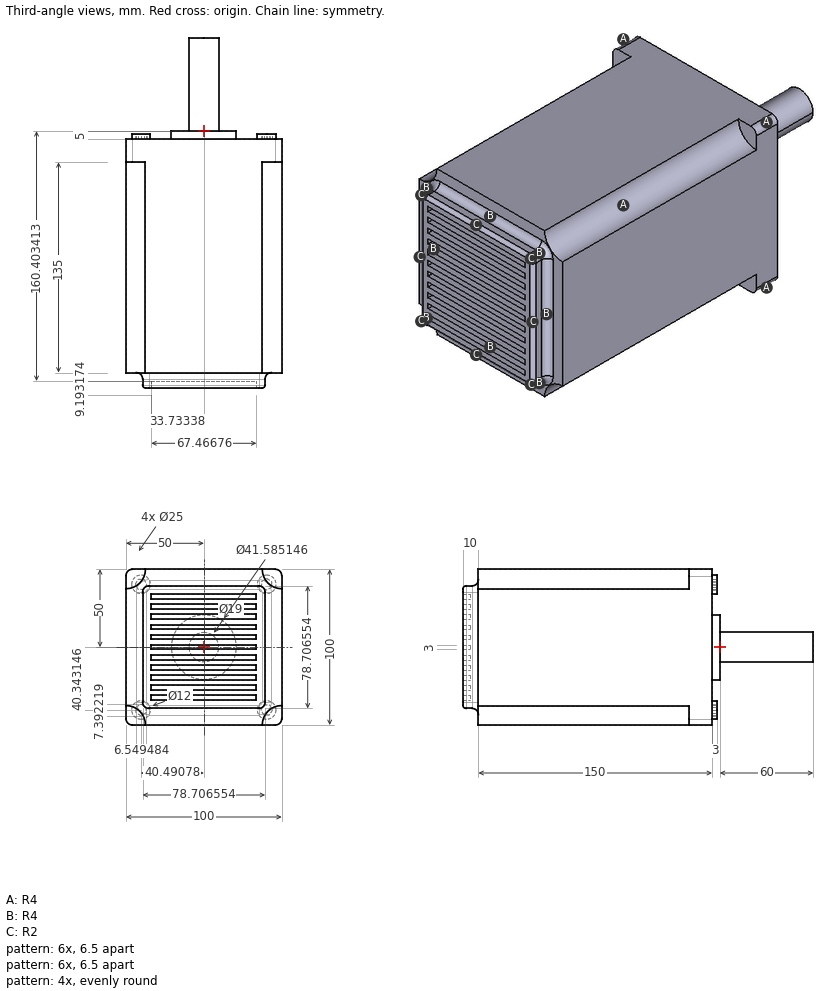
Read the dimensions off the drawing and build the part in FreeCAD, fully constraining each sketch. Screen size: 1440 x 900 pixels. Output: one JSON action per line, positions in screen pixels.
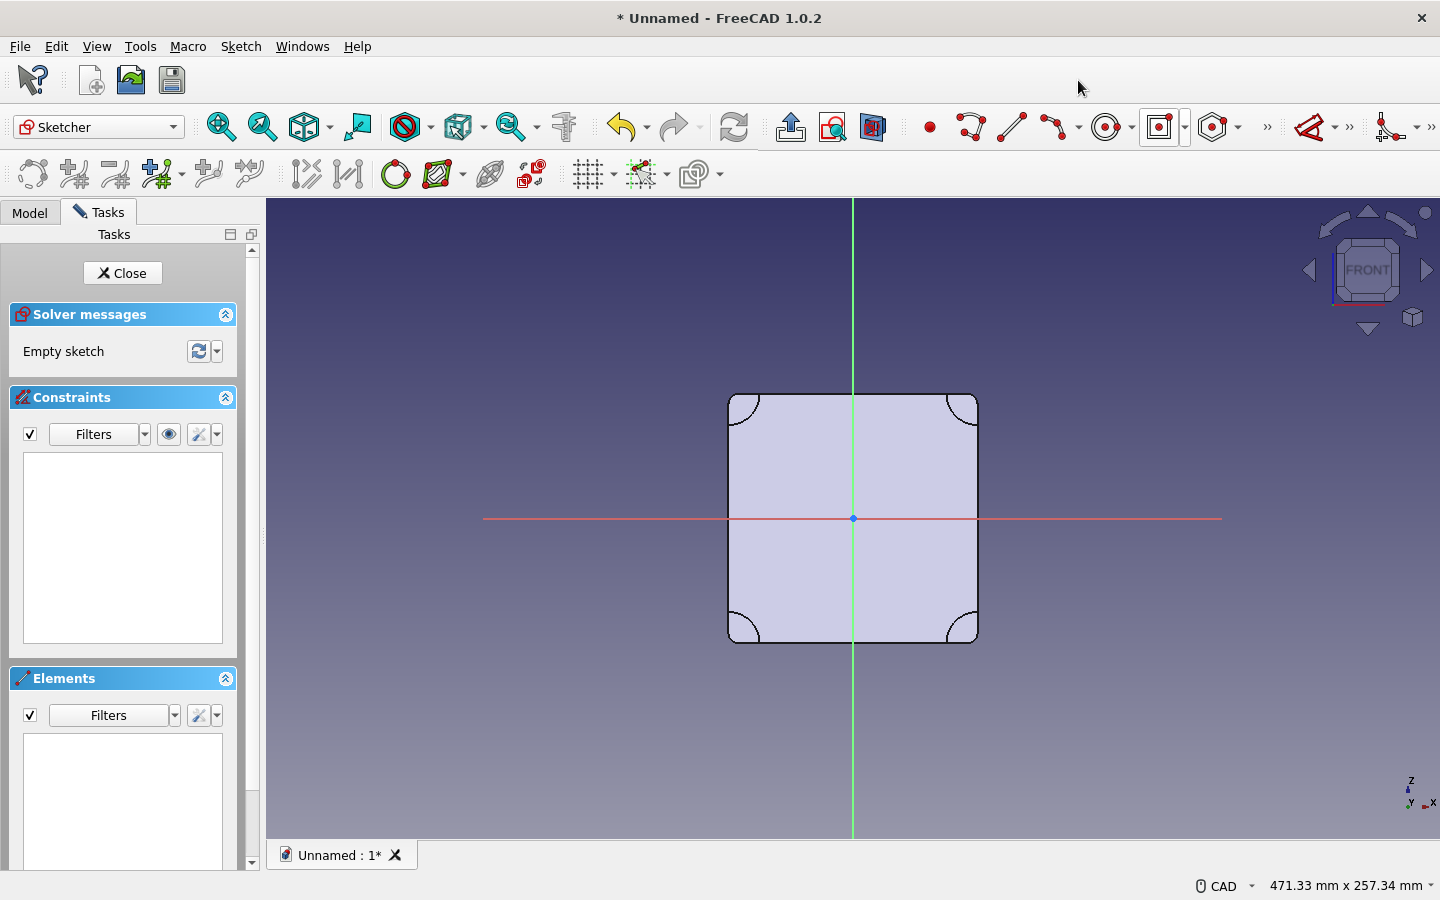
{"action": "scroll", "coordinate": [909, 518], "scroll_direction": "up", "scroll_amount": 4}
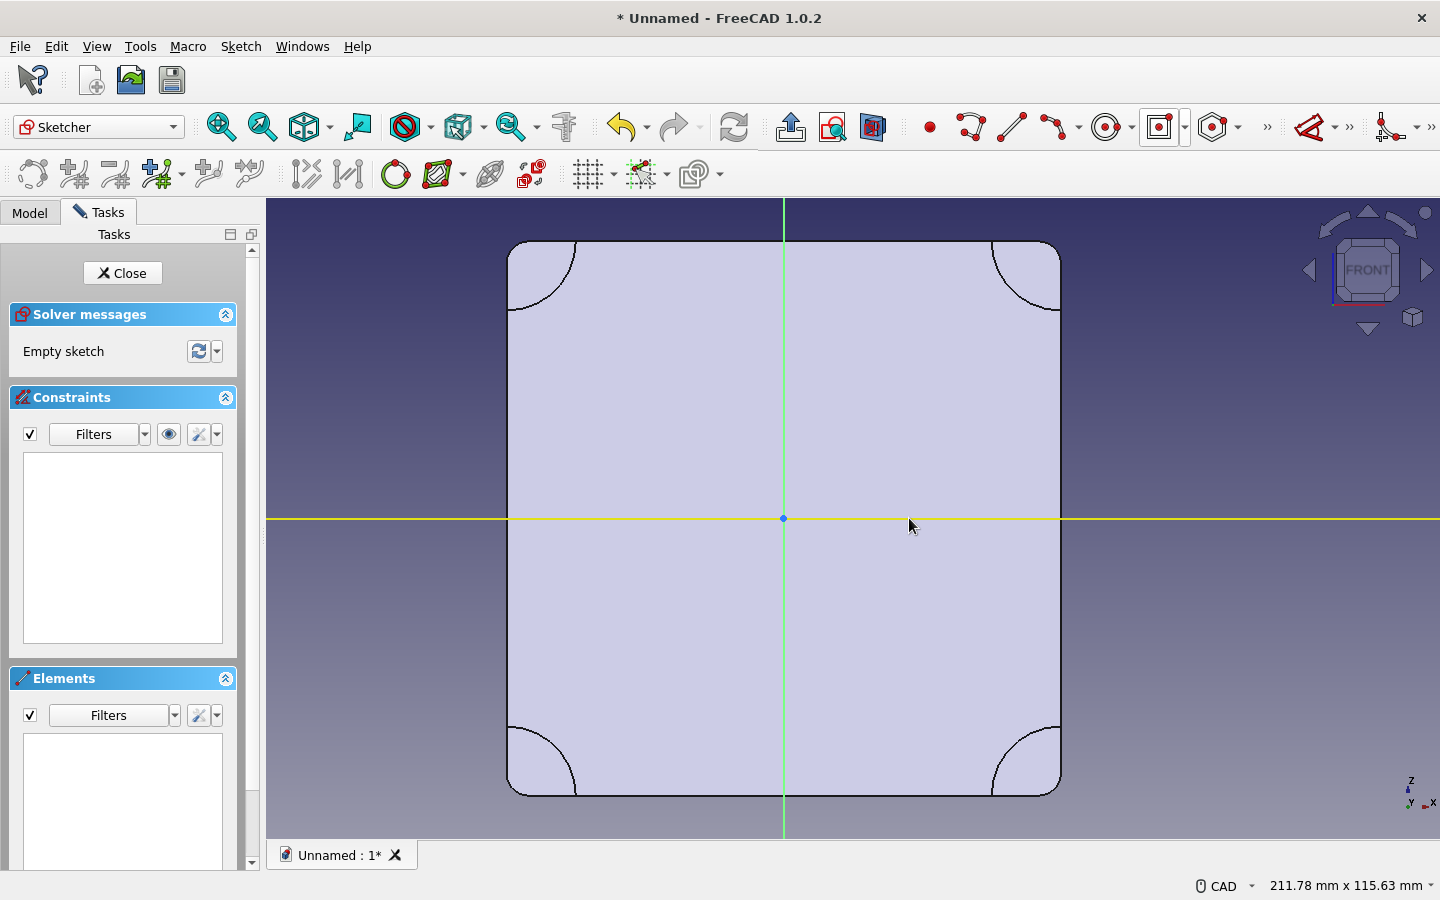
{"action": "left_click", "coordinate": [1158, 128]}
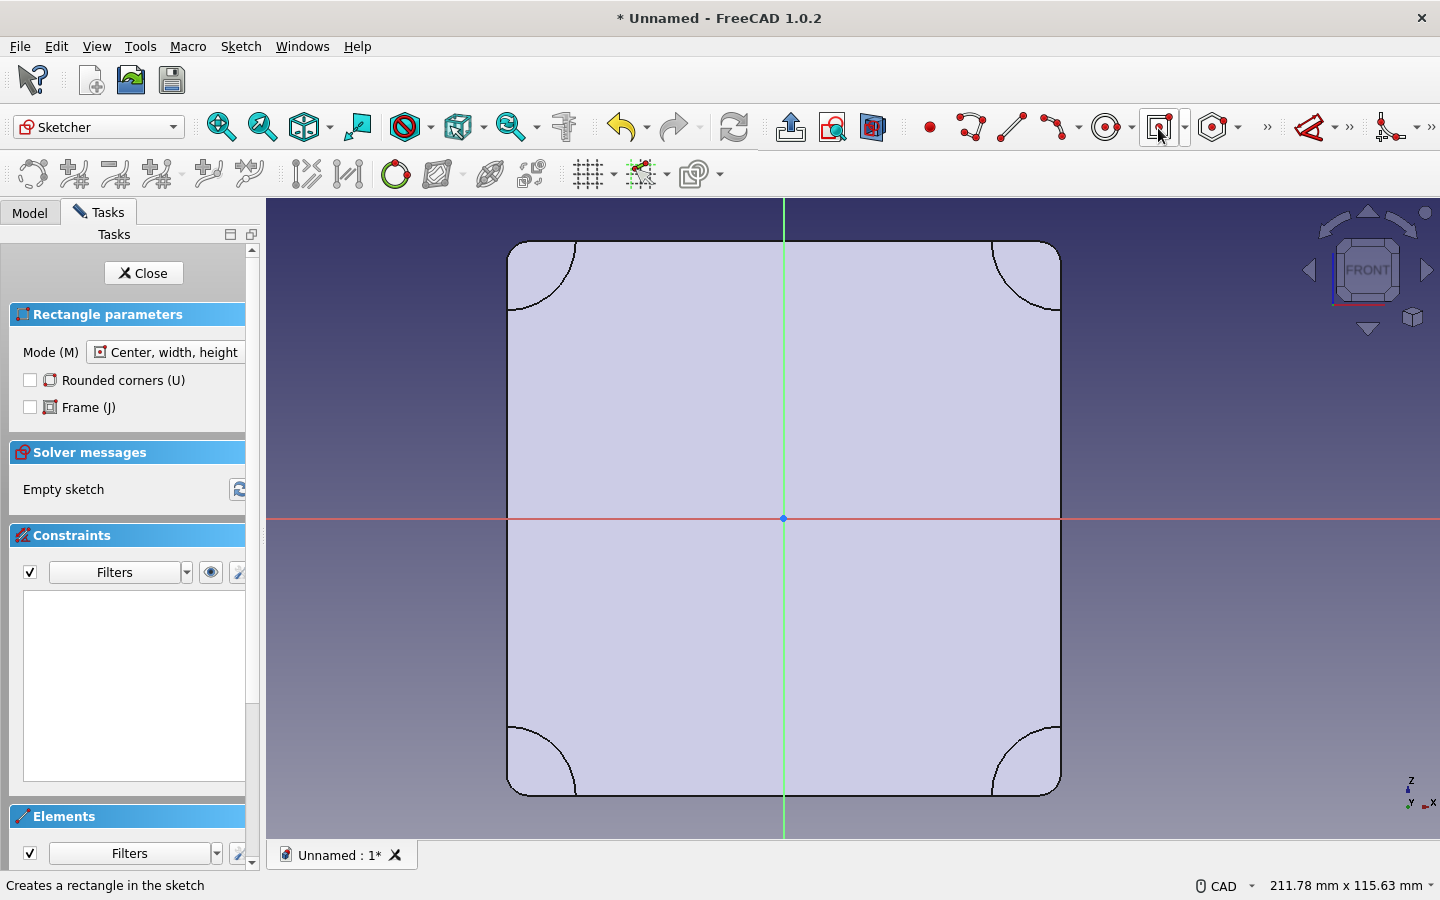
{"action": "left_click", "coordinate": [784, 518]}
{"action": "left_click", "coordinate": [1002, 300]}
{"action": "key", "text": "Escape"}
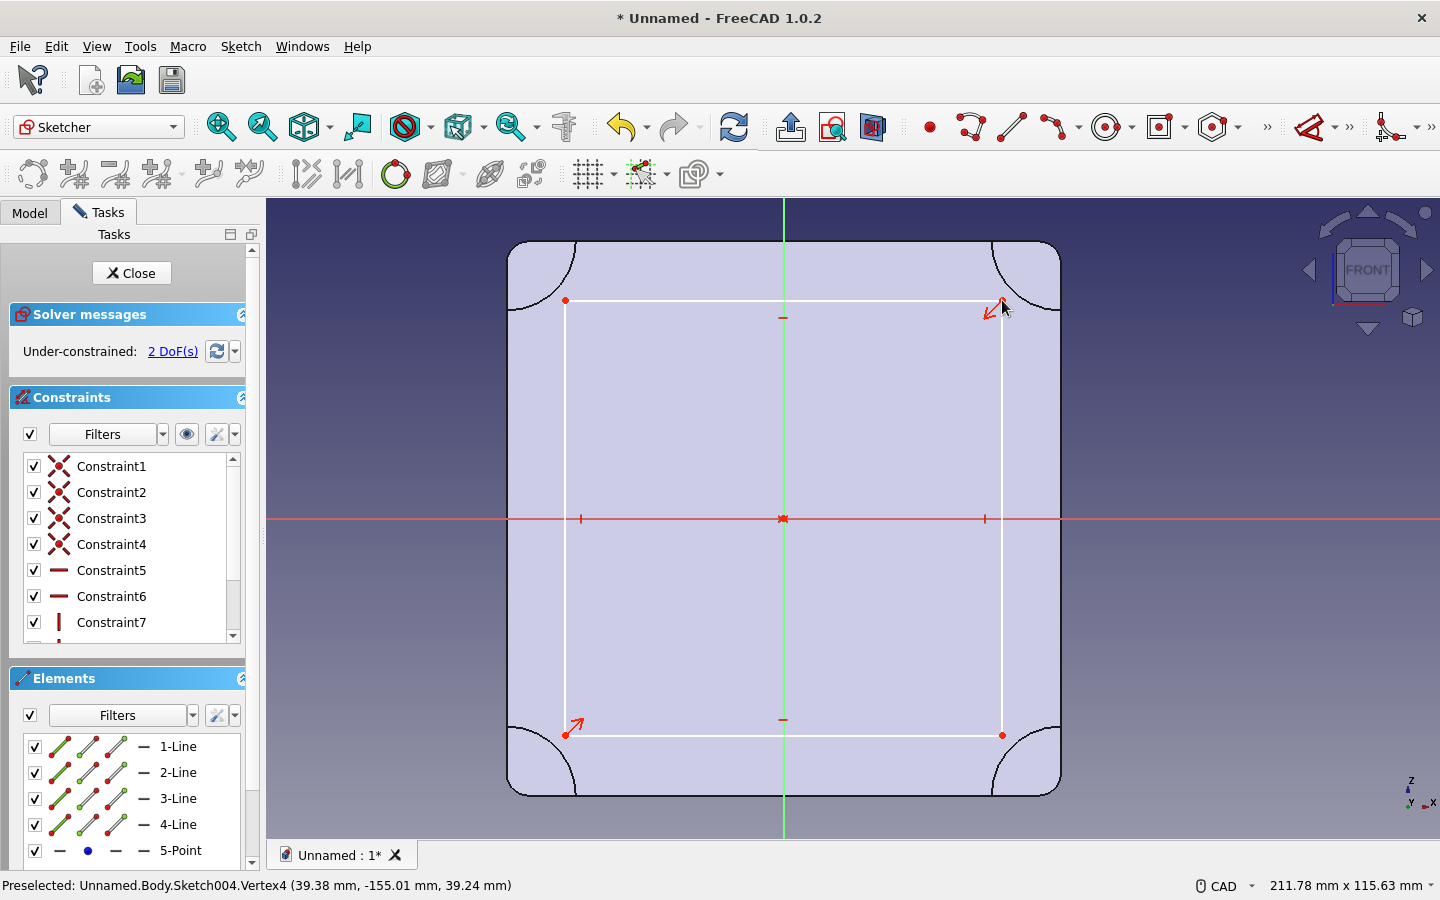
{"action": "key", "text": "d"}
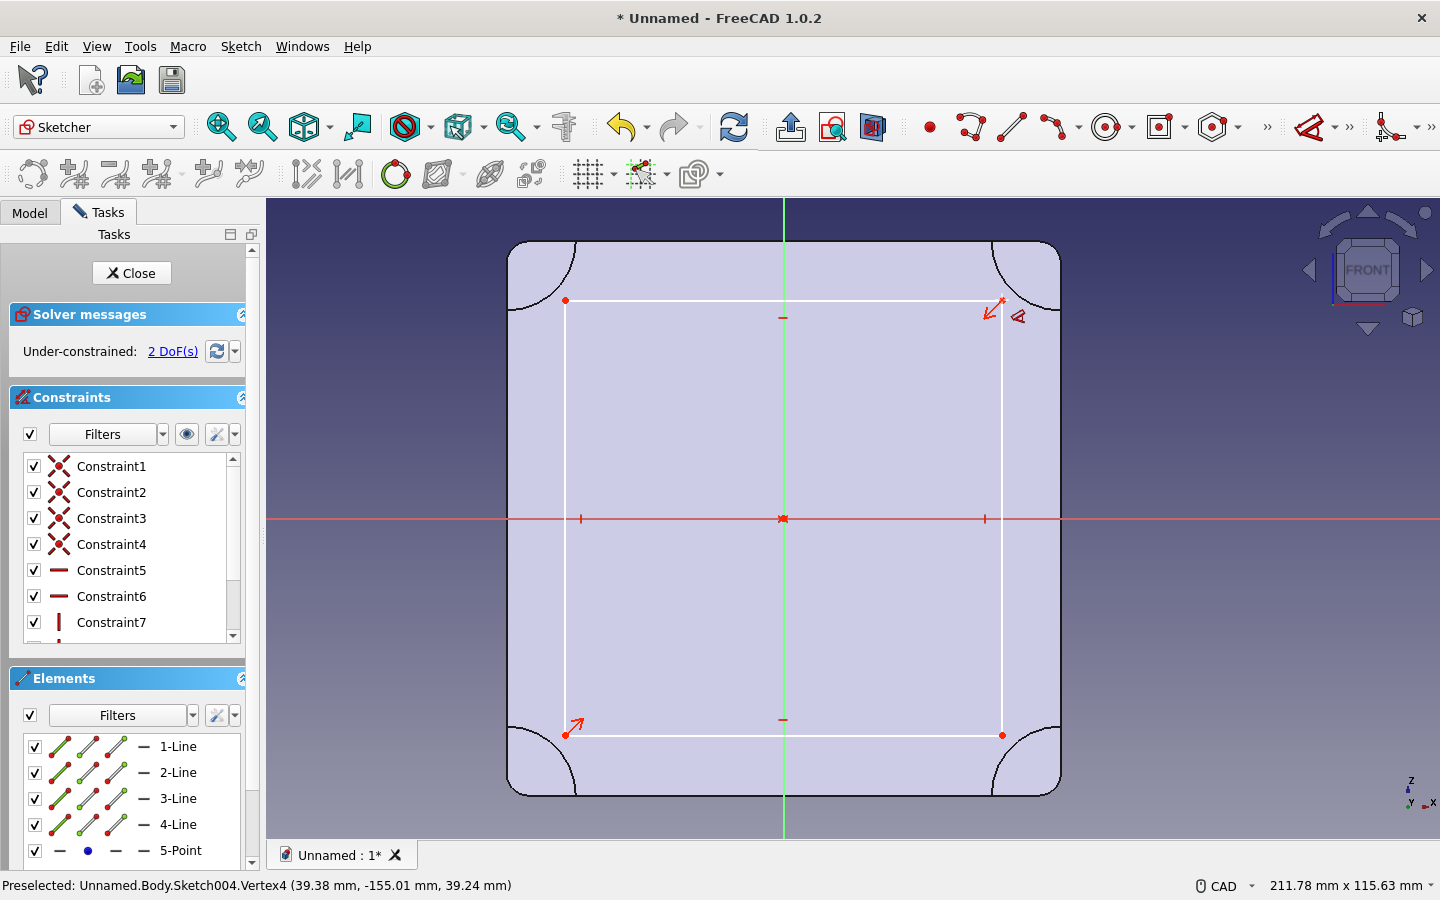
{"action": "left_click", "coordinate": [696, 736]}
{"action": "left_click", "coordinate": [683, 770]}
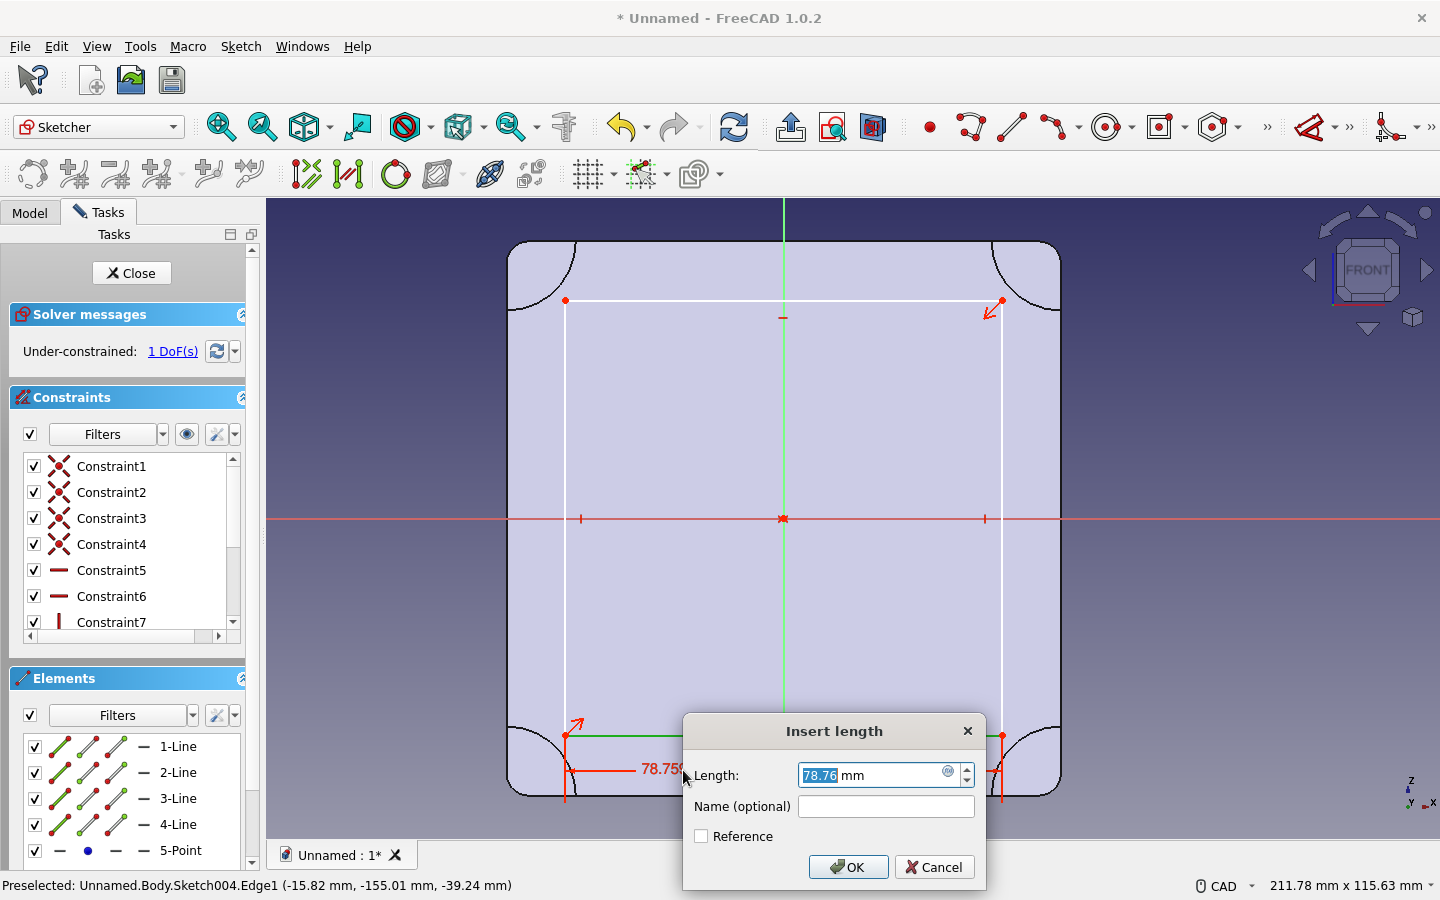
{"action": "type", "text": "78.706554"}
{"action": "key", "text": "Return"}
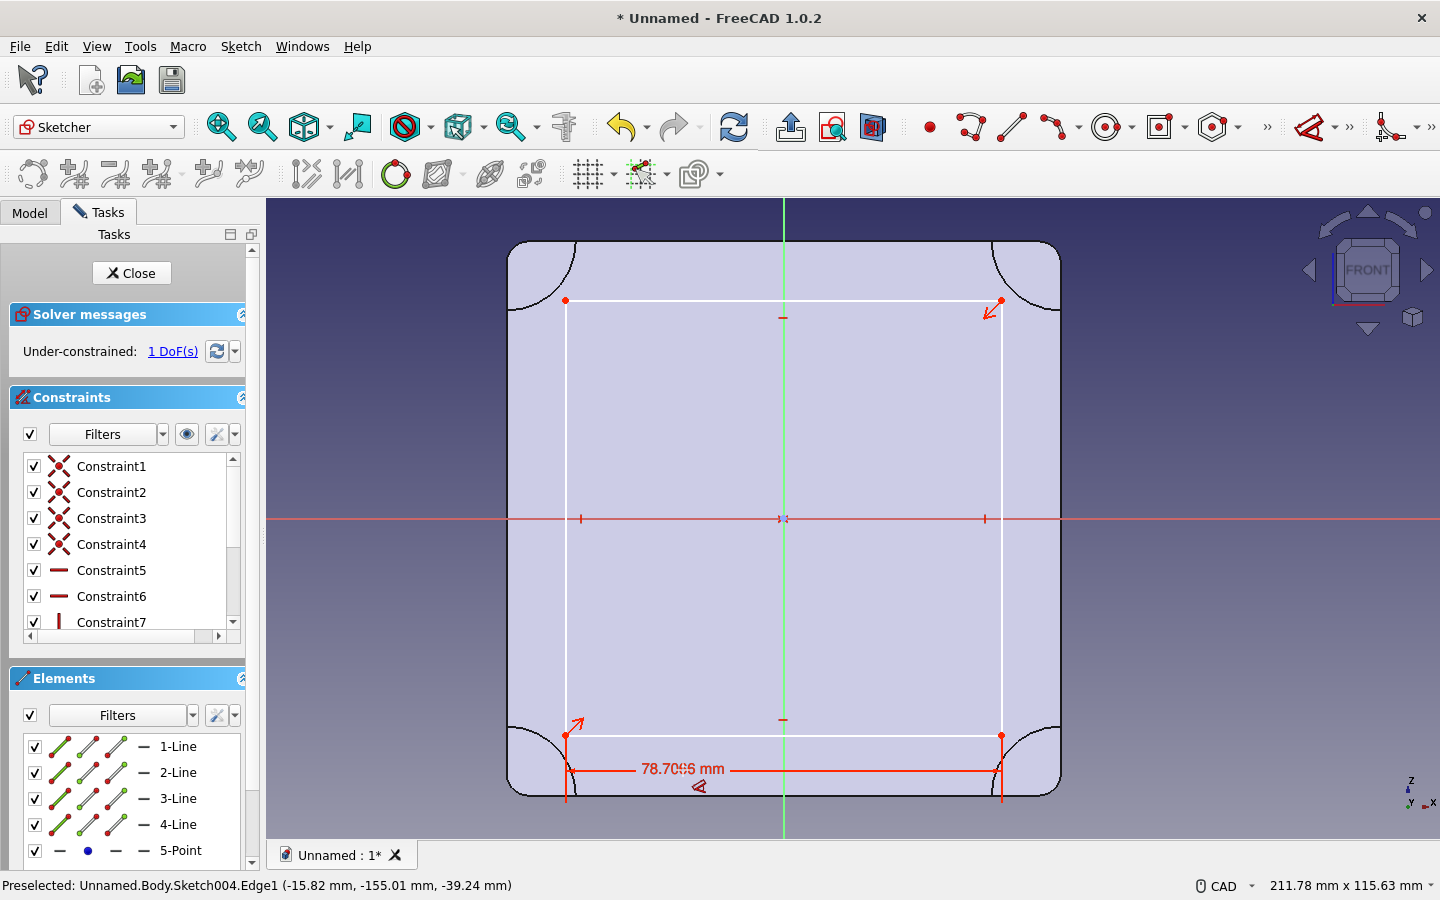
{"action": "left_click", "coordinate": [1002, 605]}
{"action": "left_click", "coordinate": [1036, 418]}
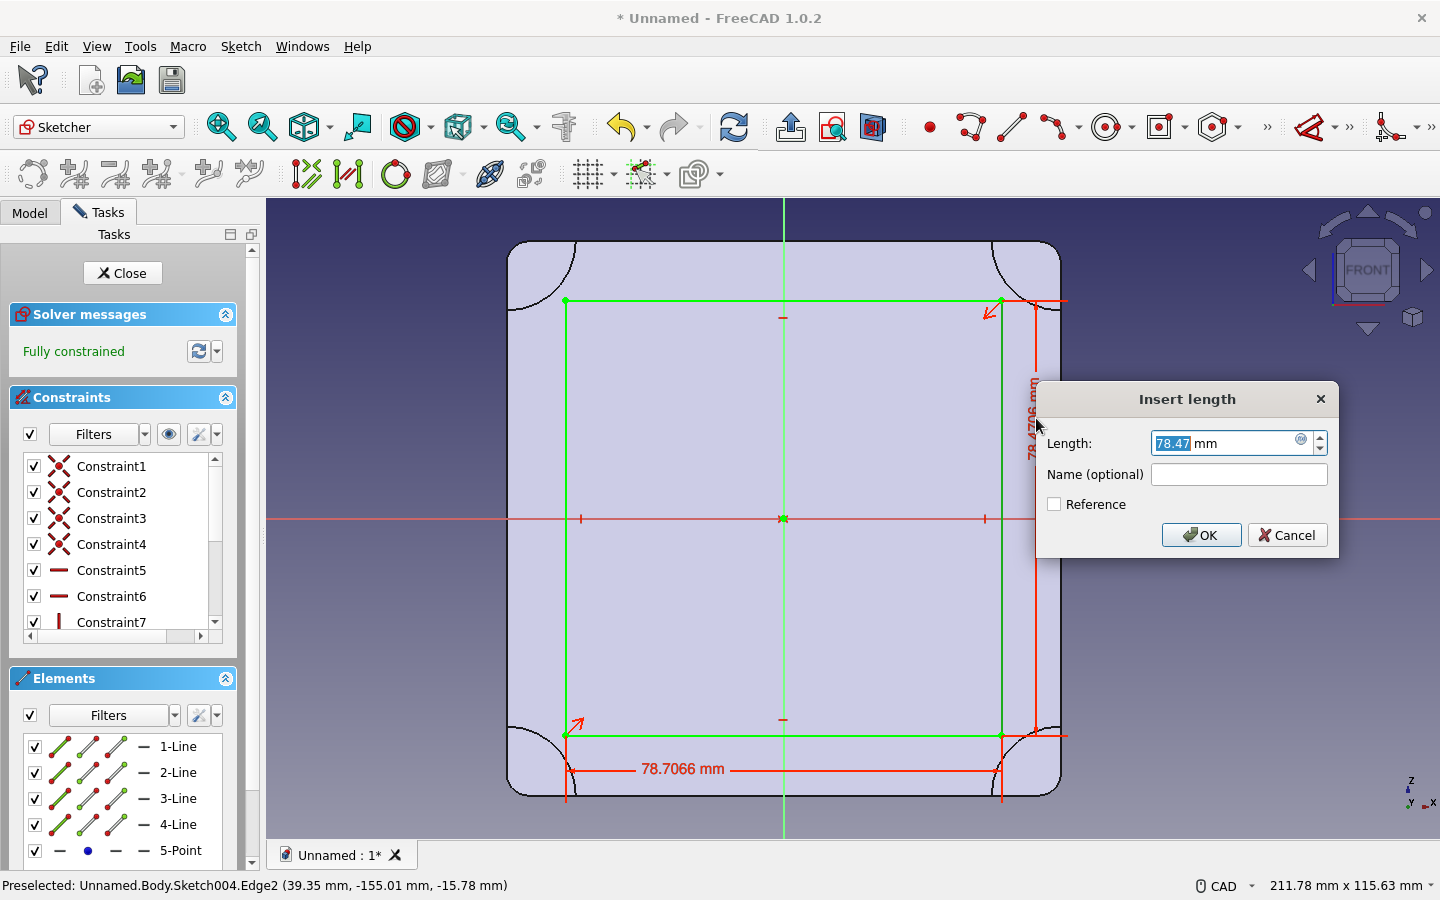
{"action": "type", "text": "78.706554"}
{"action": "key", "text": "Return"}
{"action": "key", "text": "Escape"}